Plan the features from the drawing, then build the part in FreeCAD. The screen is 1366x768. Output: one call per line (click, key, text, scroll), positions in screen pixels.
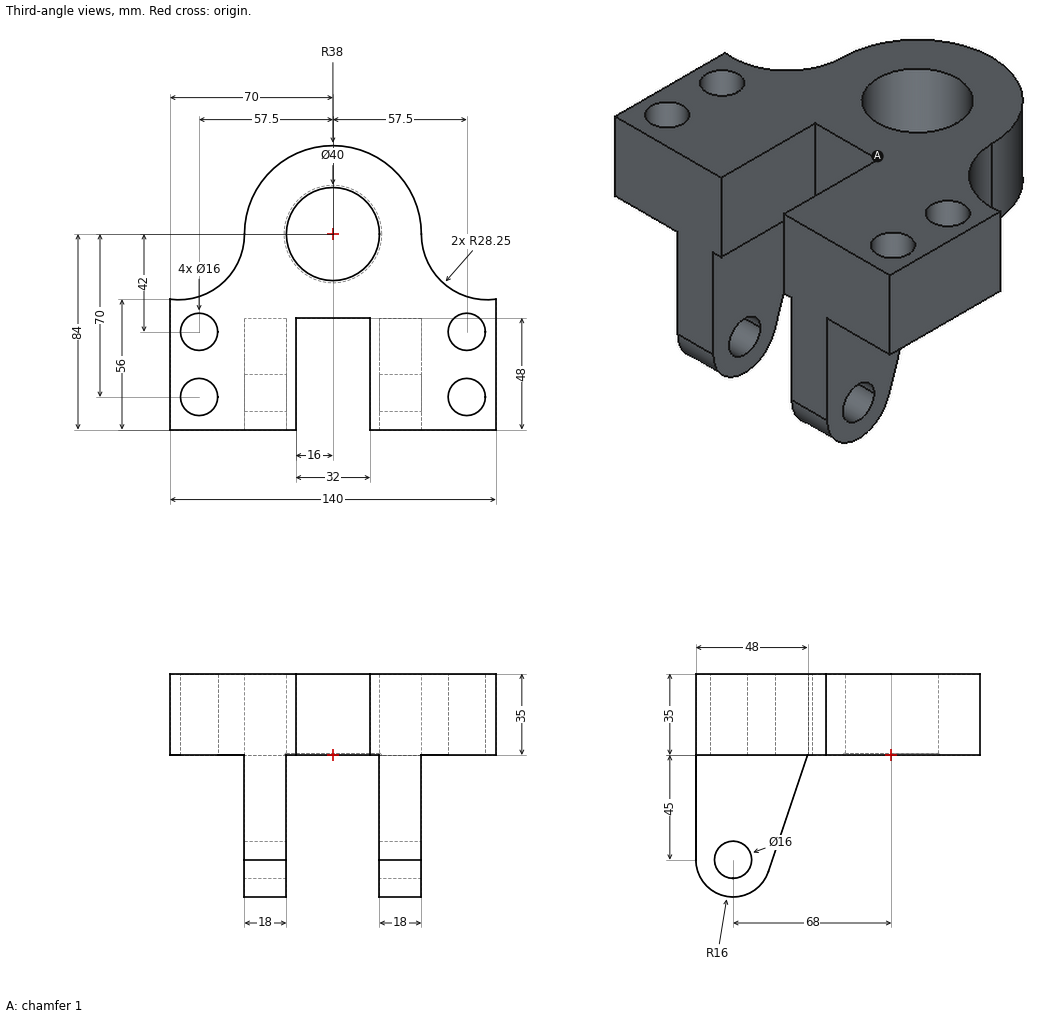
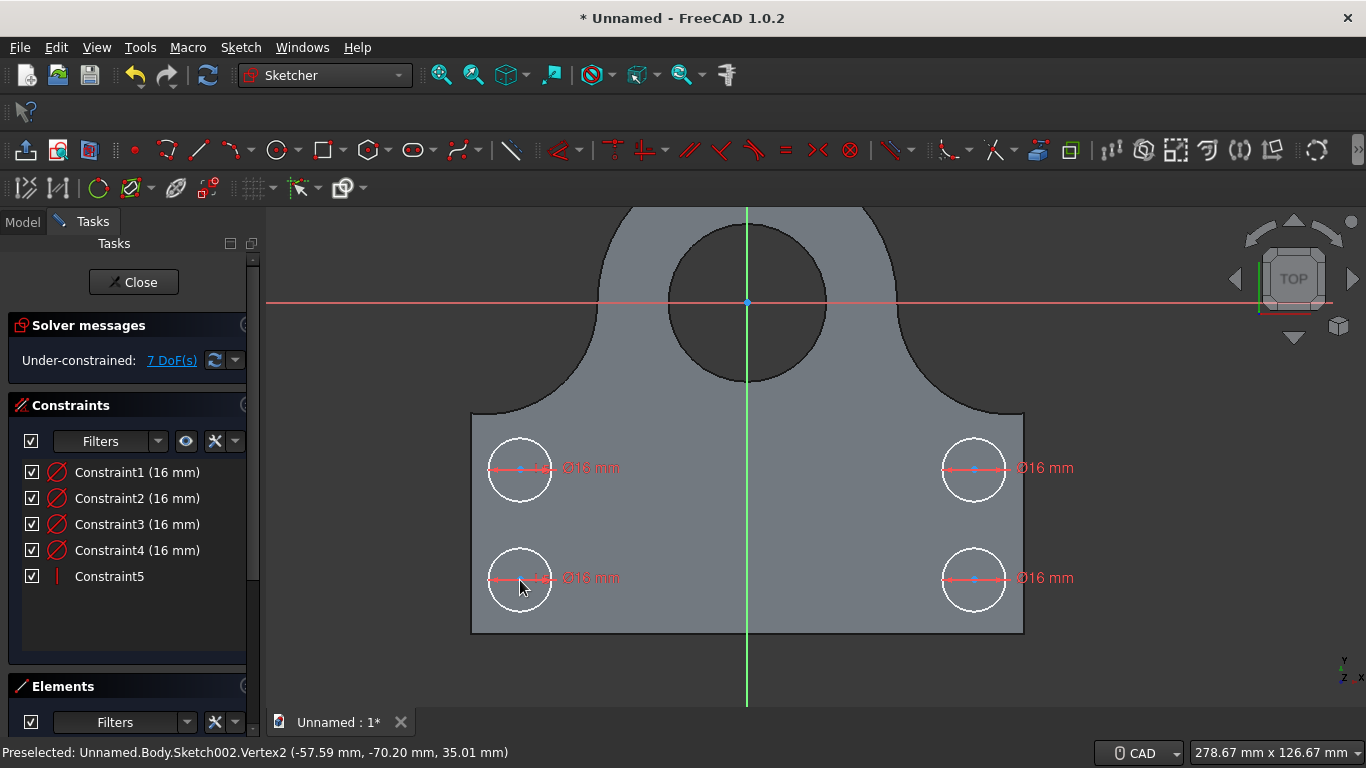
click(520, 470)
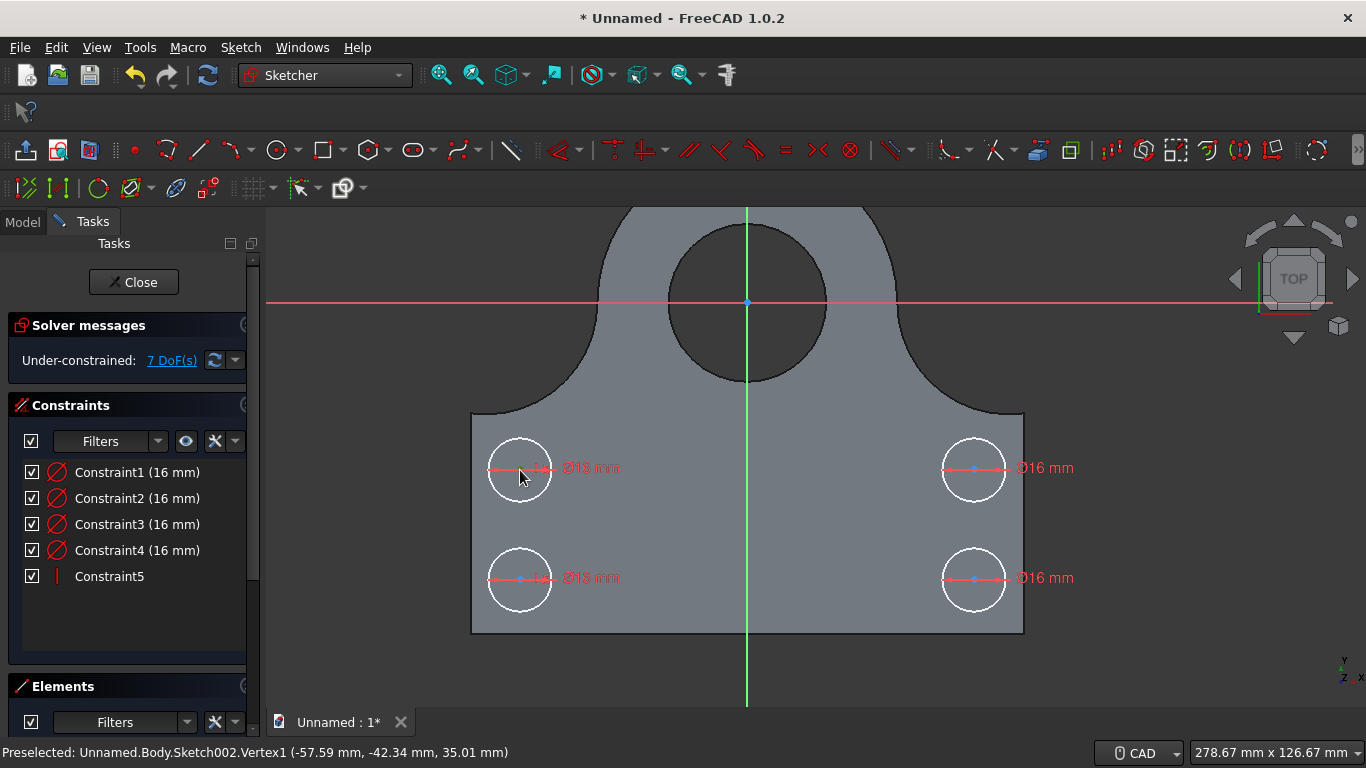
click(974, 470)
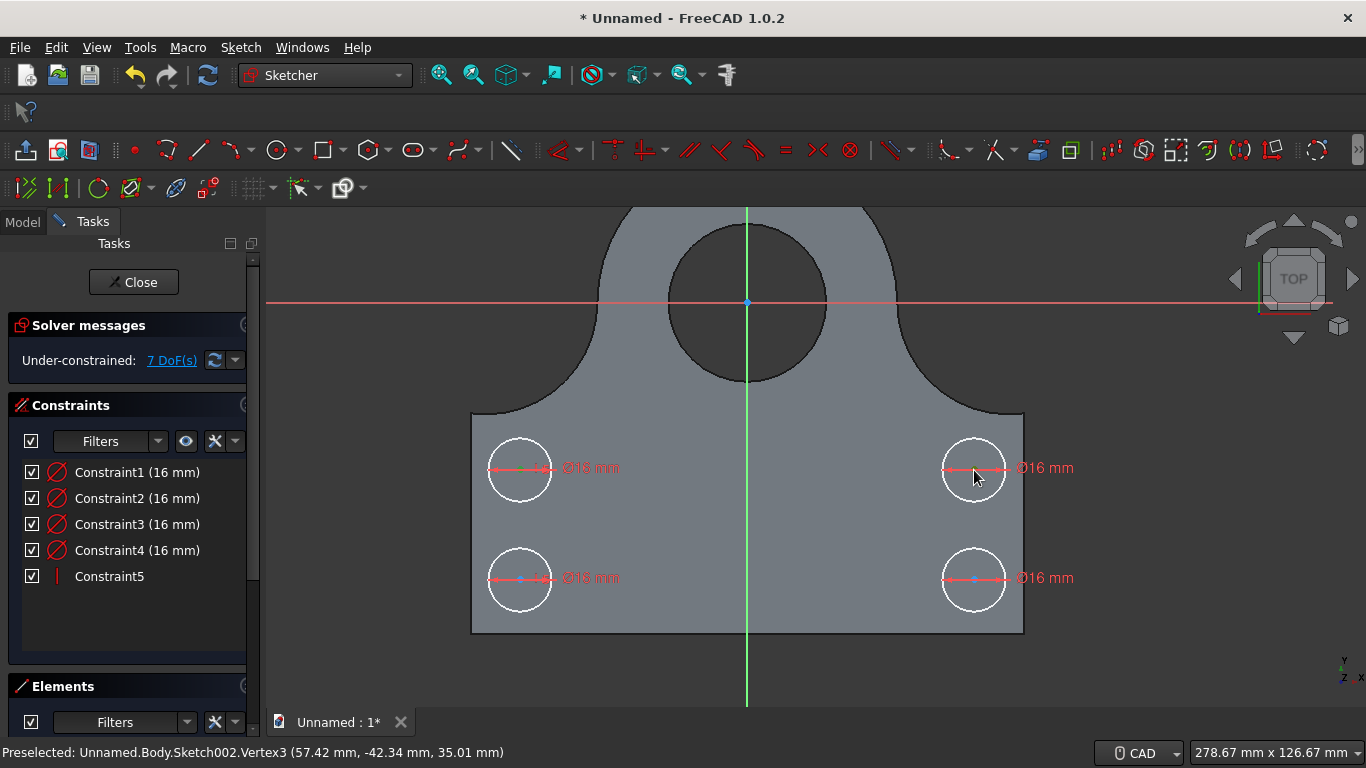
key(h)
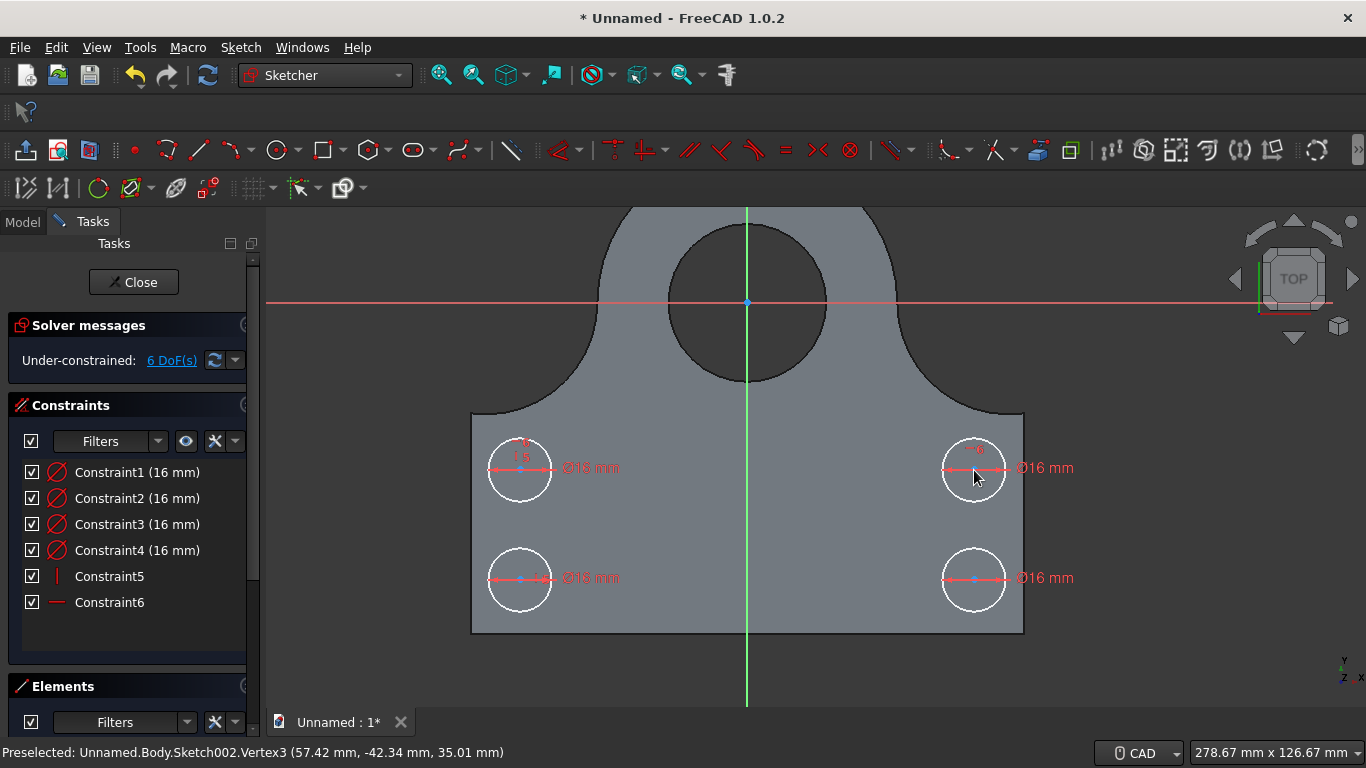
click(974, 470)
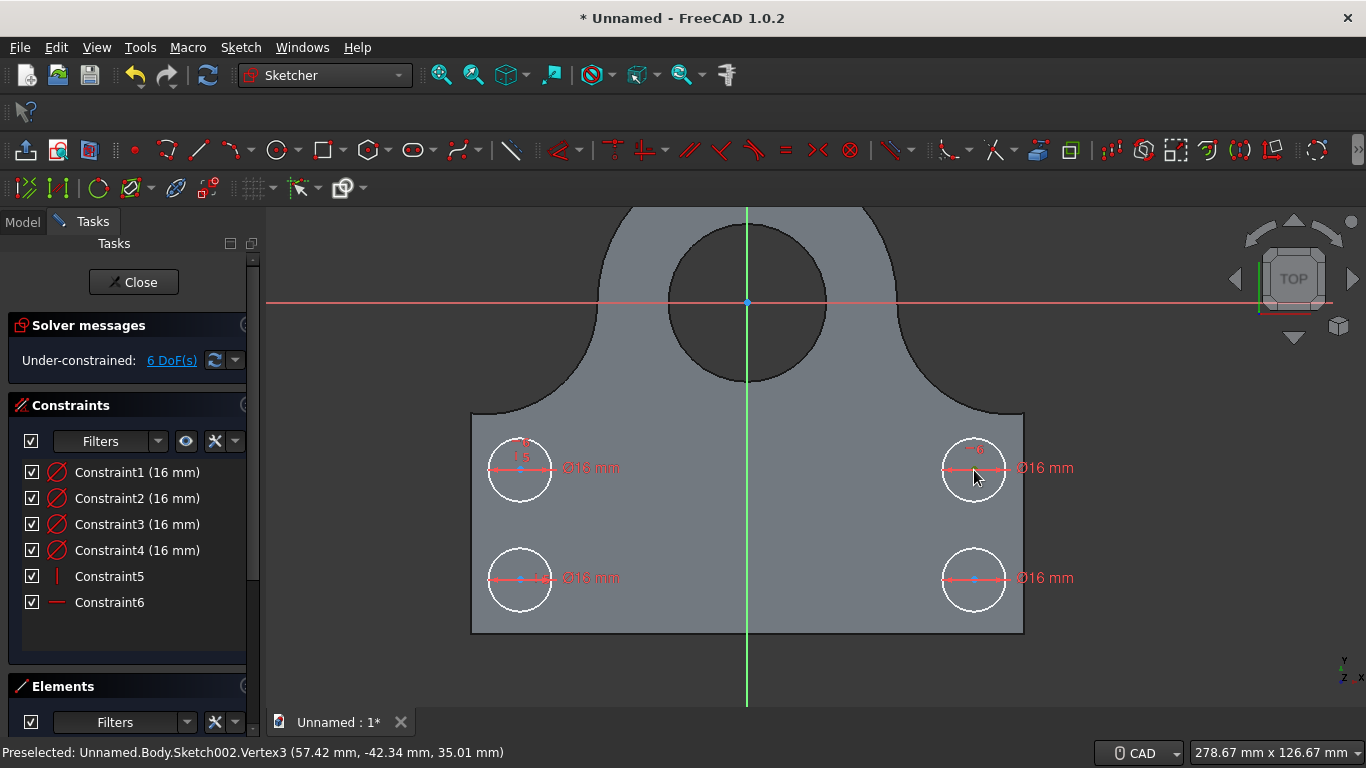
click(974, 580)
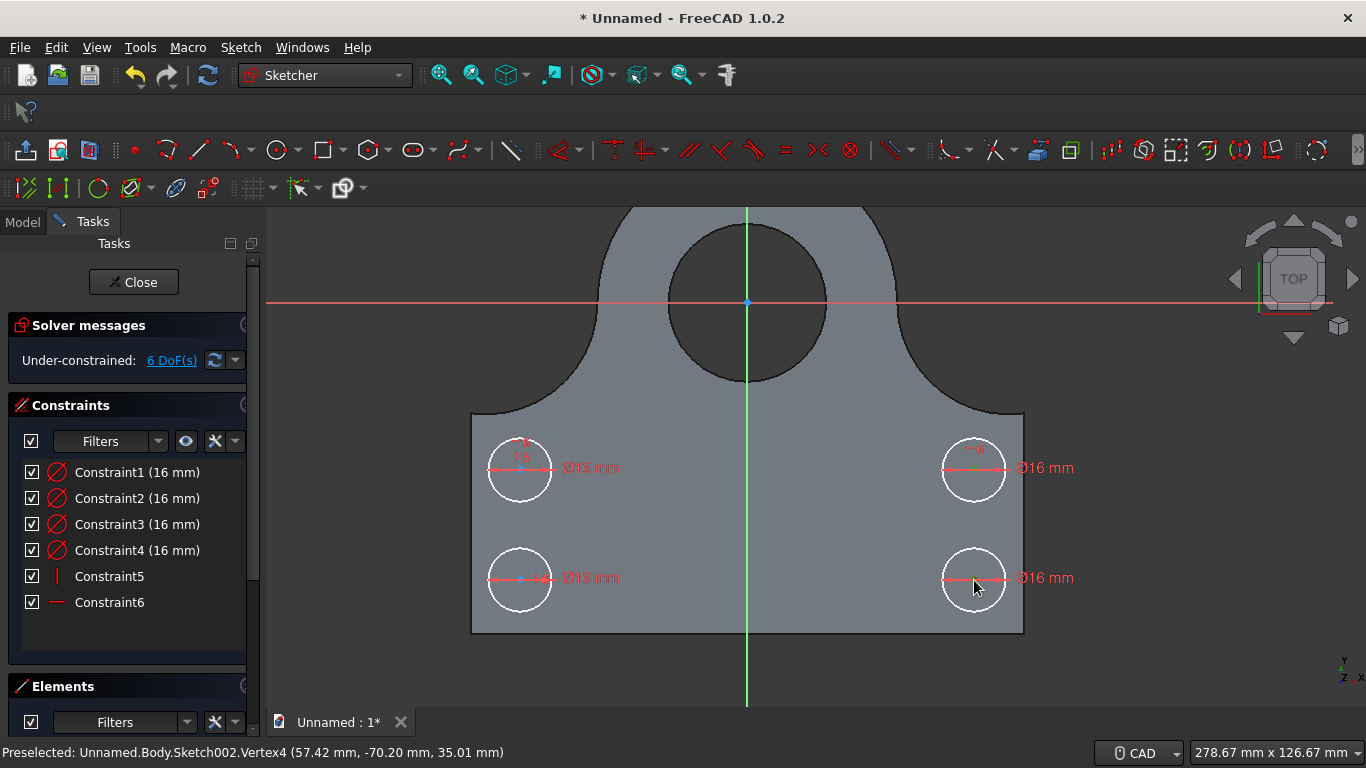
key(v)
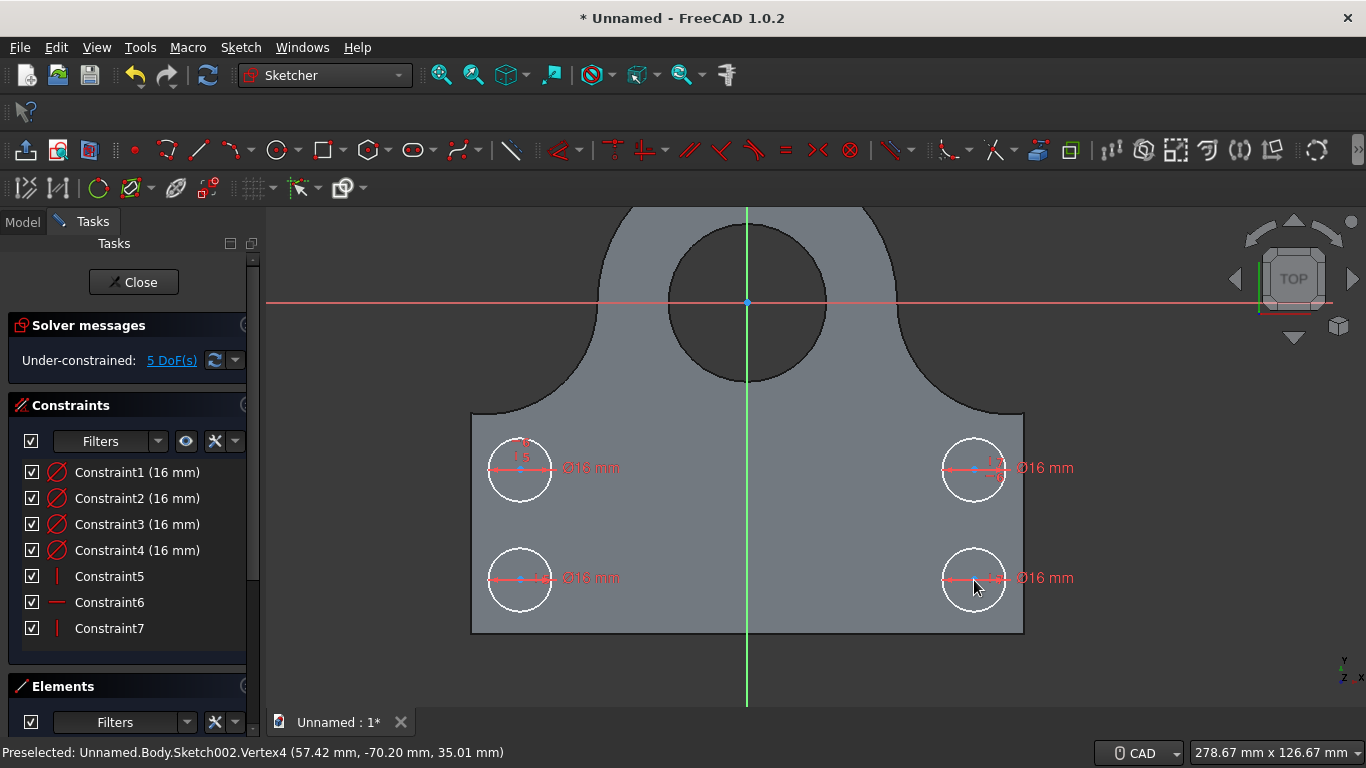
click(520, 580)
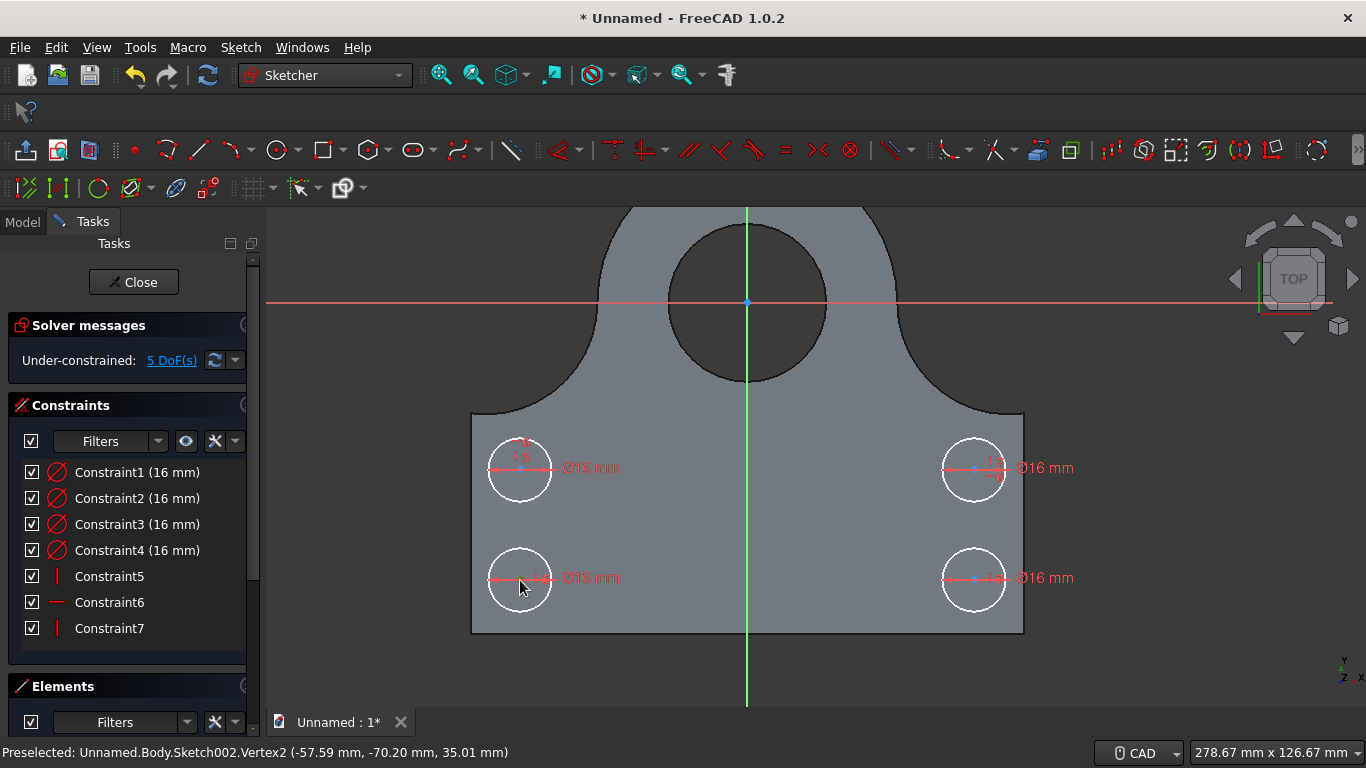
click(974, 580)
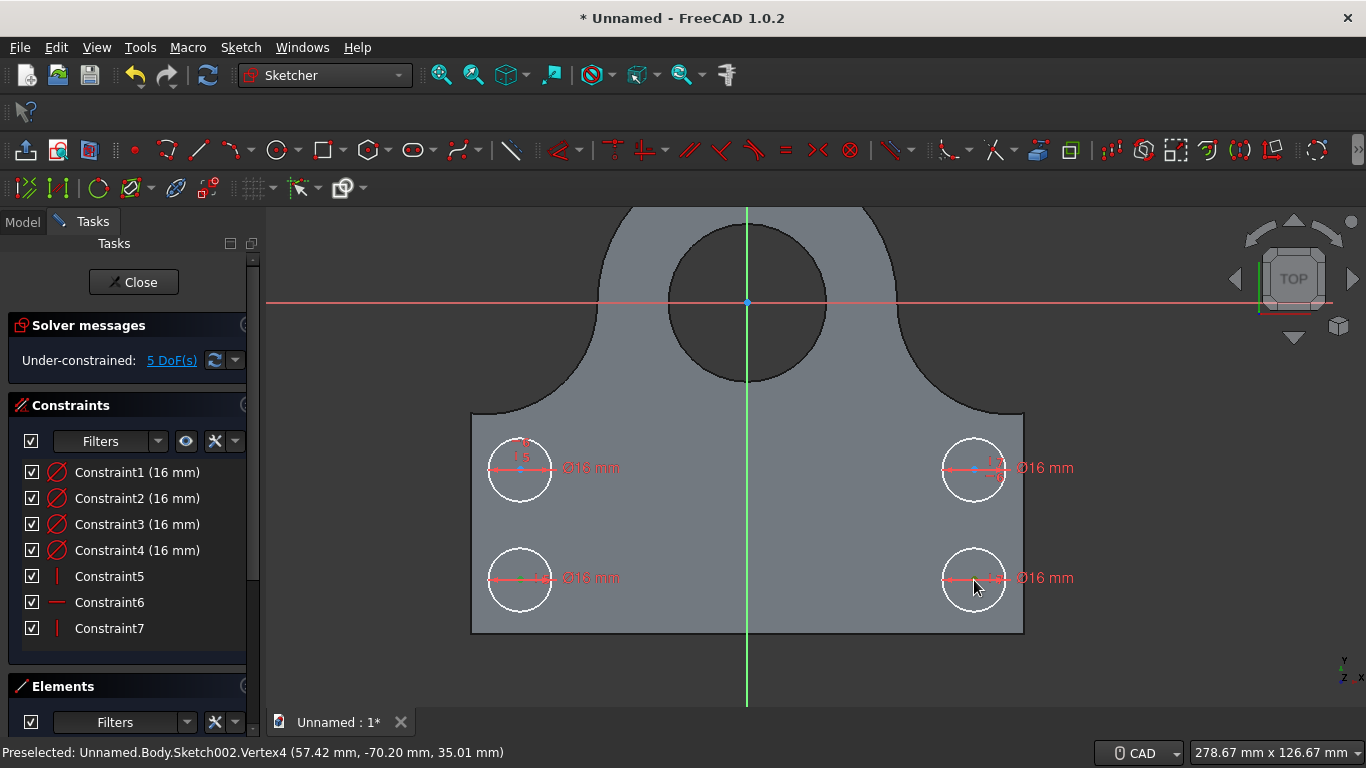
key(h)